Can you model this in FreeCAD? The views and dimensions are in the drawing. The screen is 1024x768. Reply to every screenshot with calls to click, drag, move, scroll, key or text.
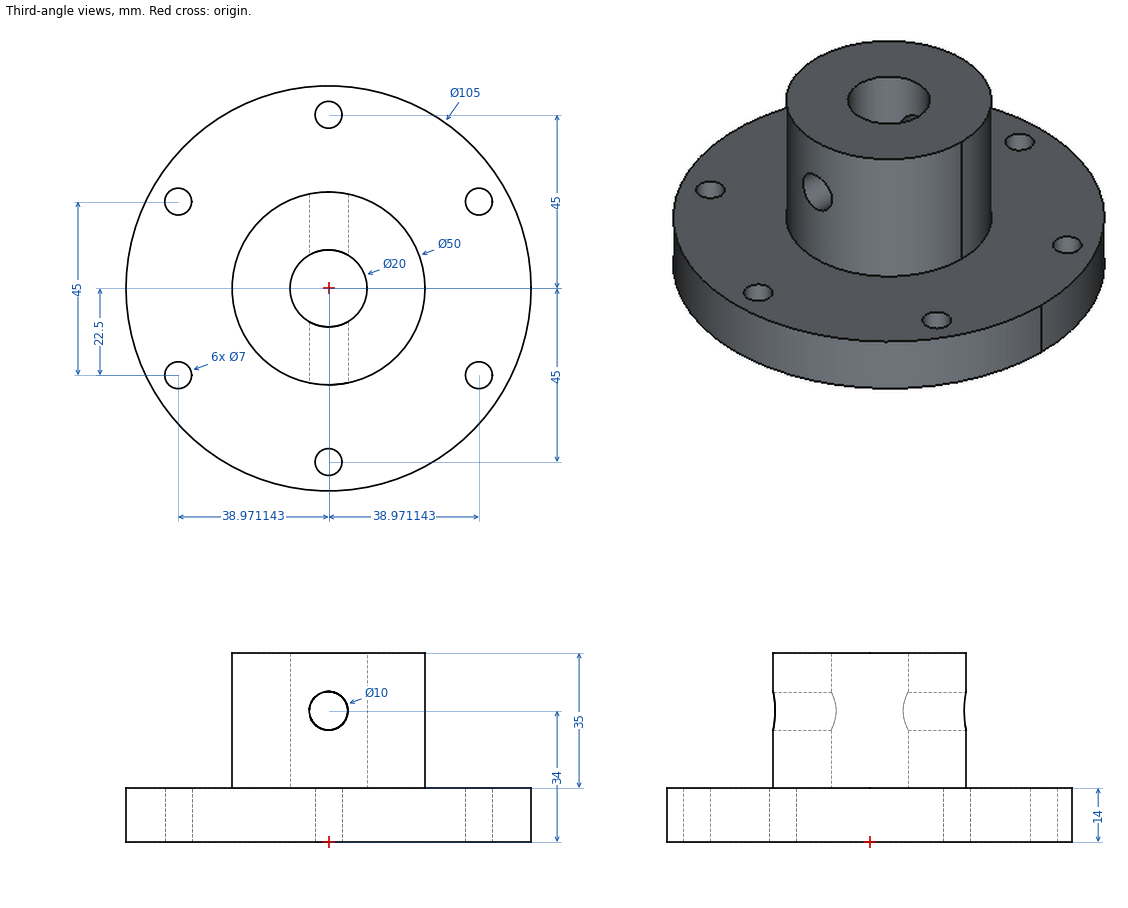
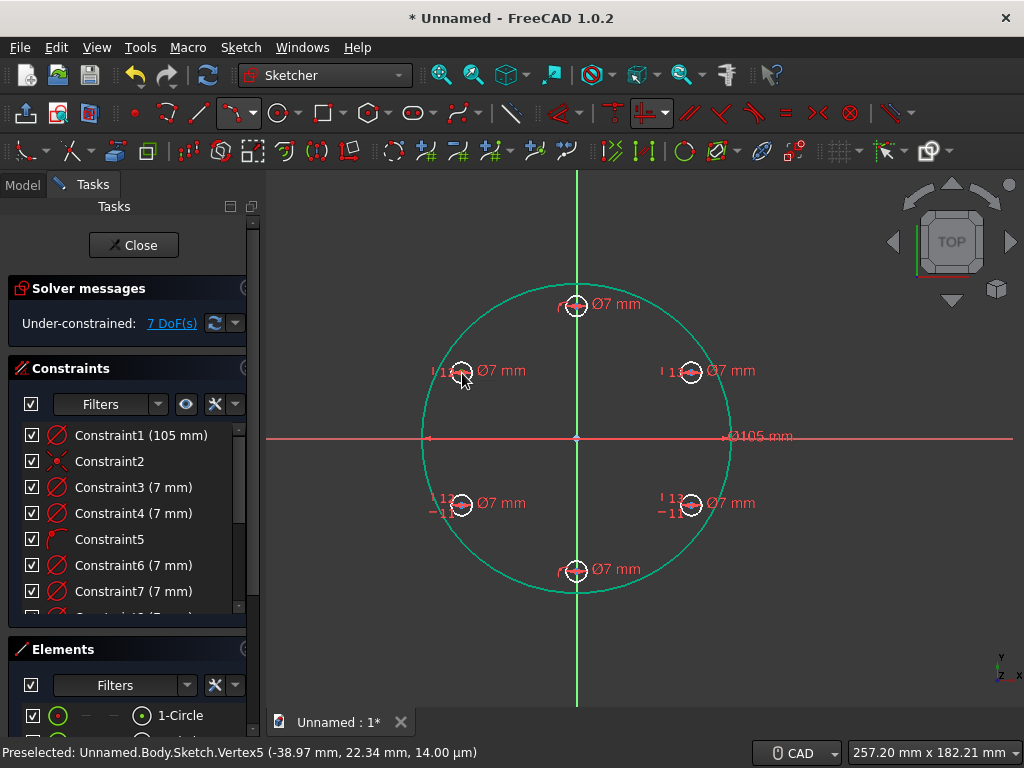
click(691, 373)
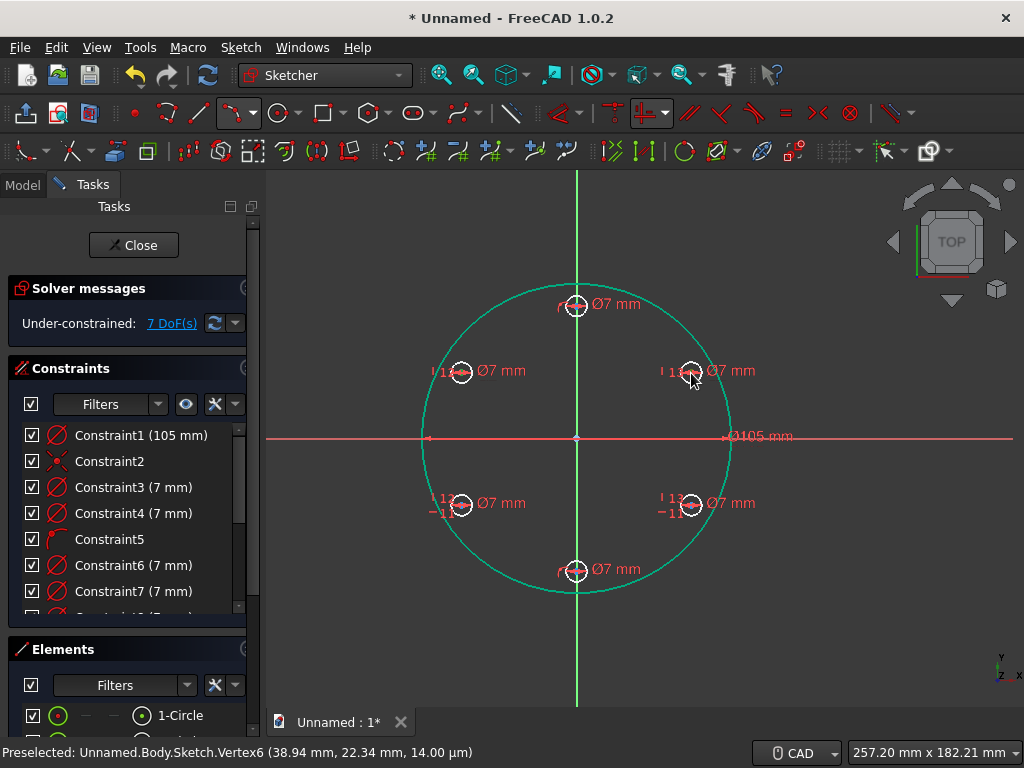
key(h)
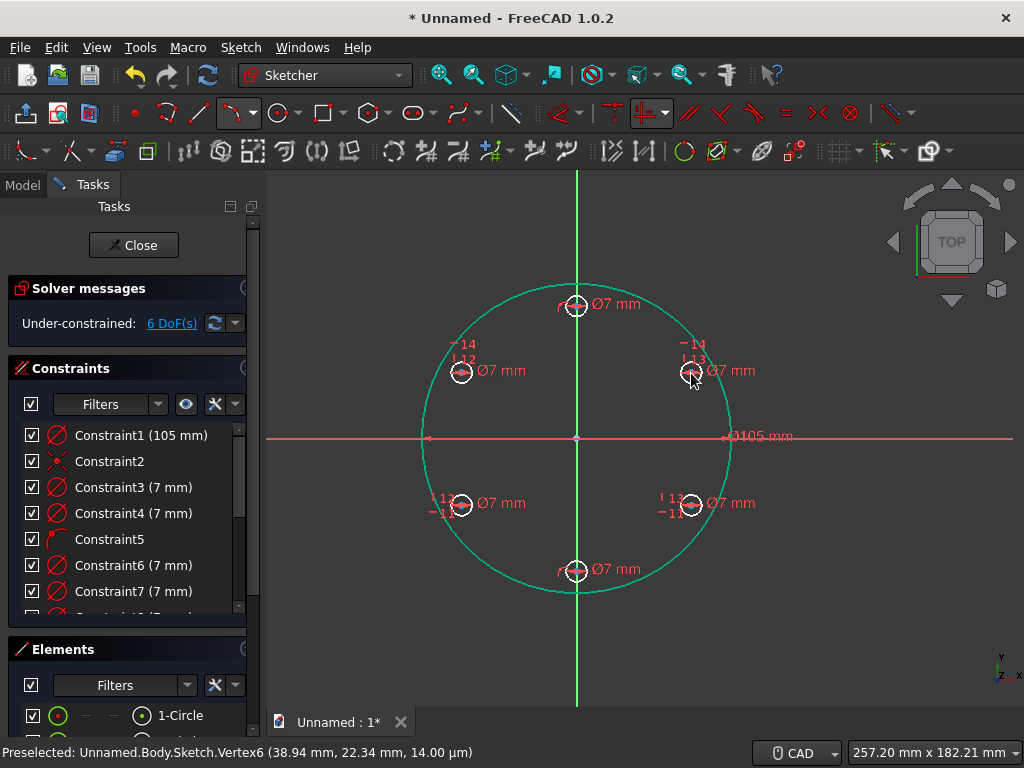
key(d)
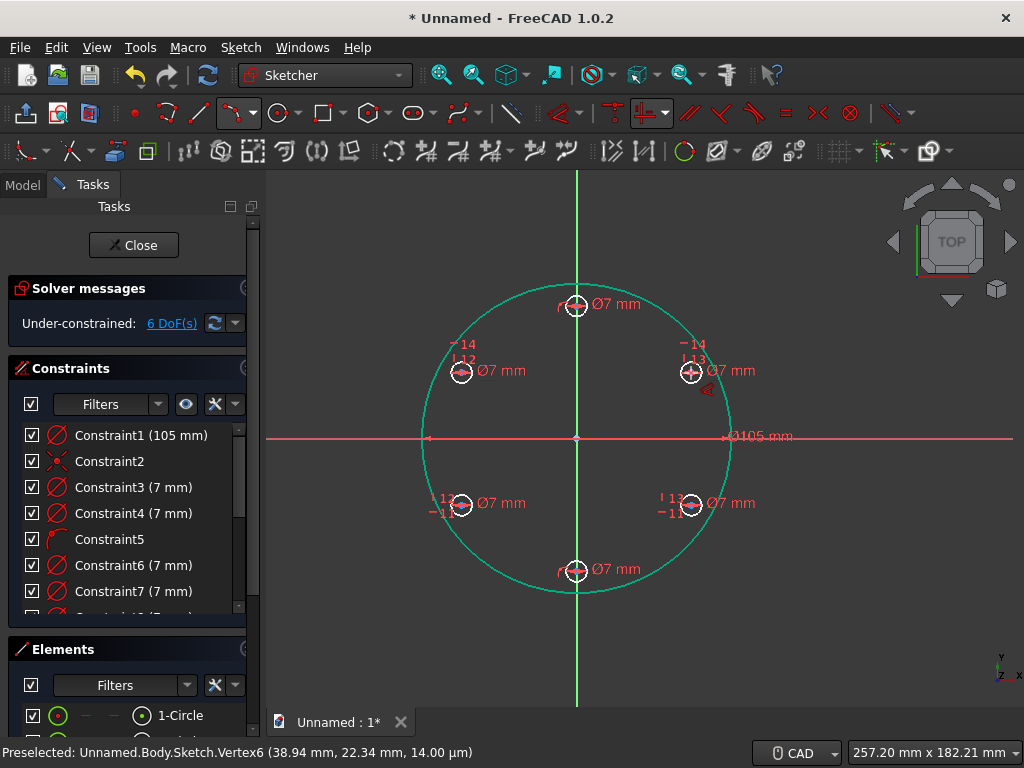
click(577, 571)
click(611, 505)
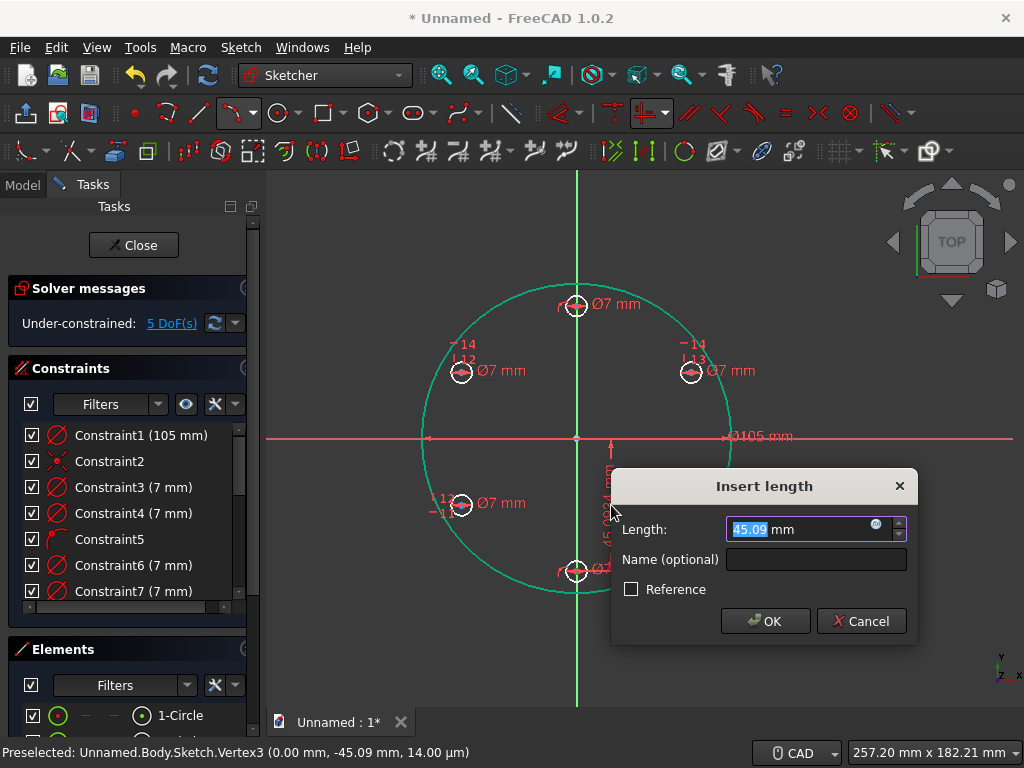
text(45)
key(Return)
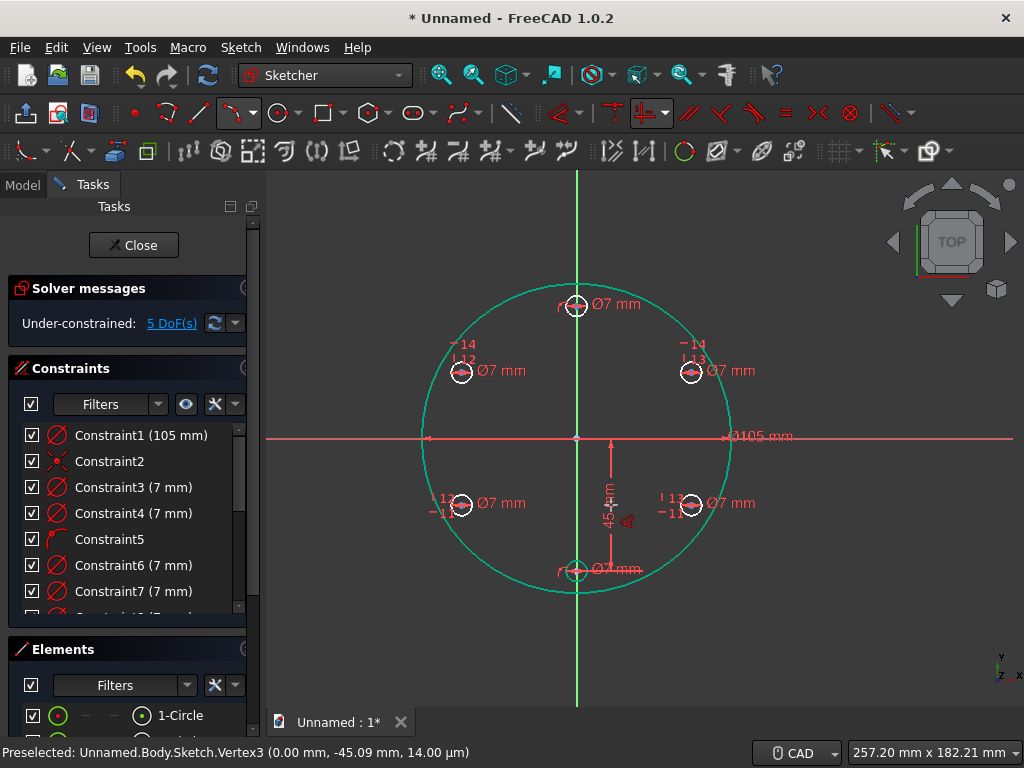
click(577, 306)
click(611, 372)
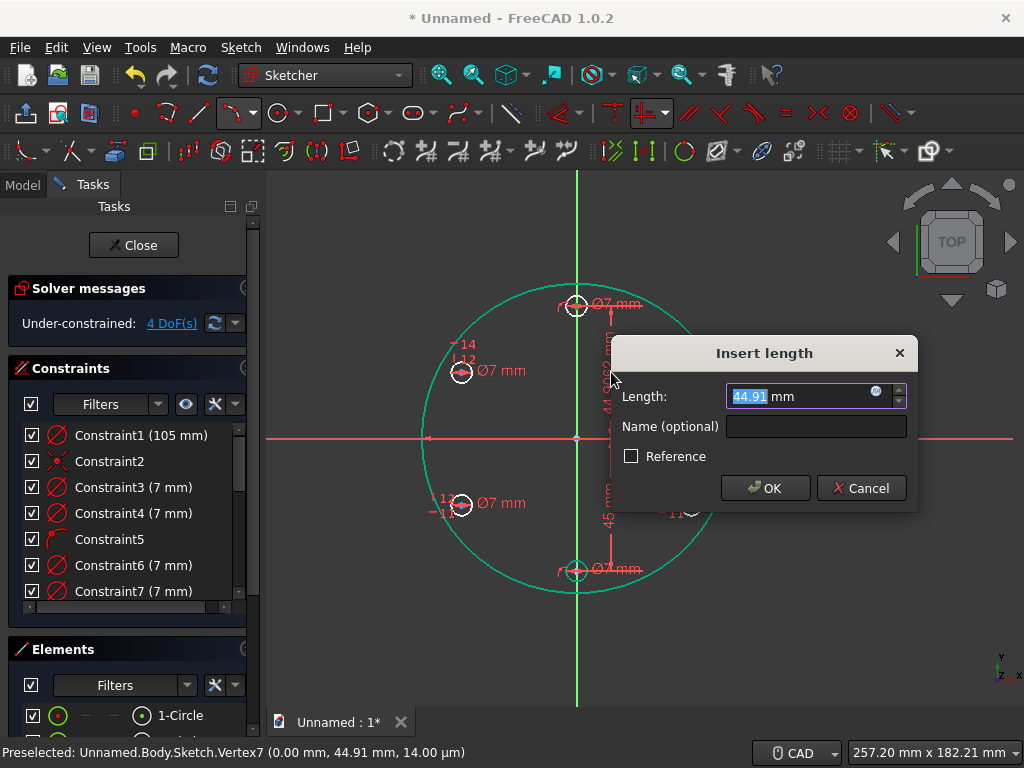
text(45)
key(Return)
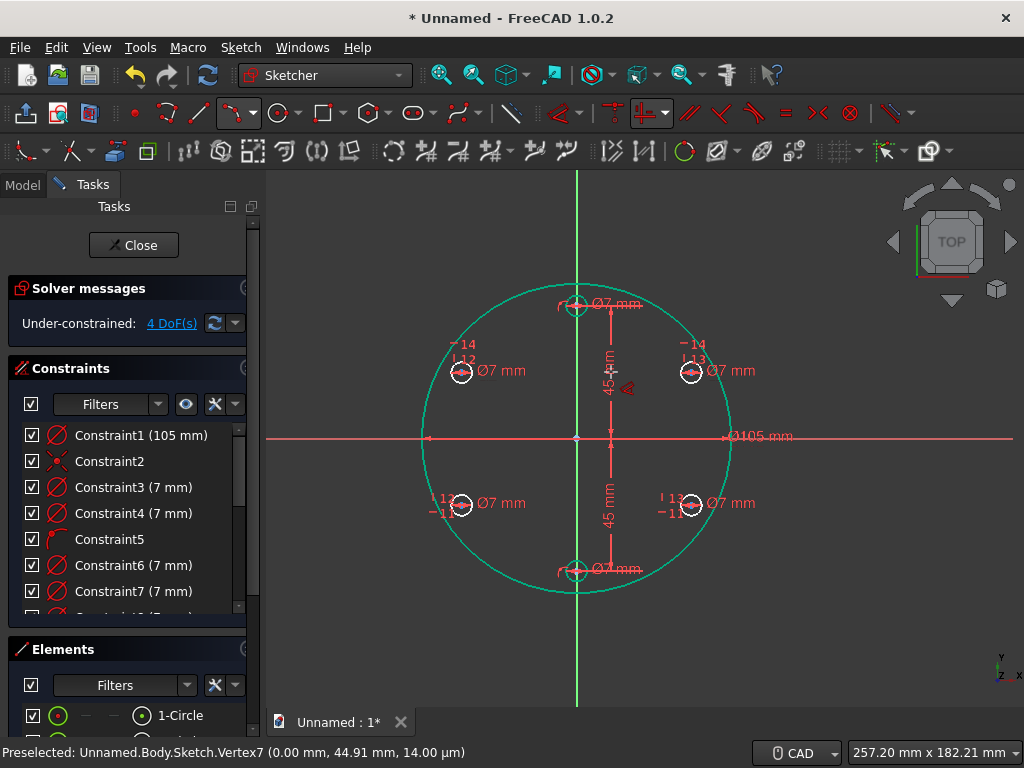
click(462, 505)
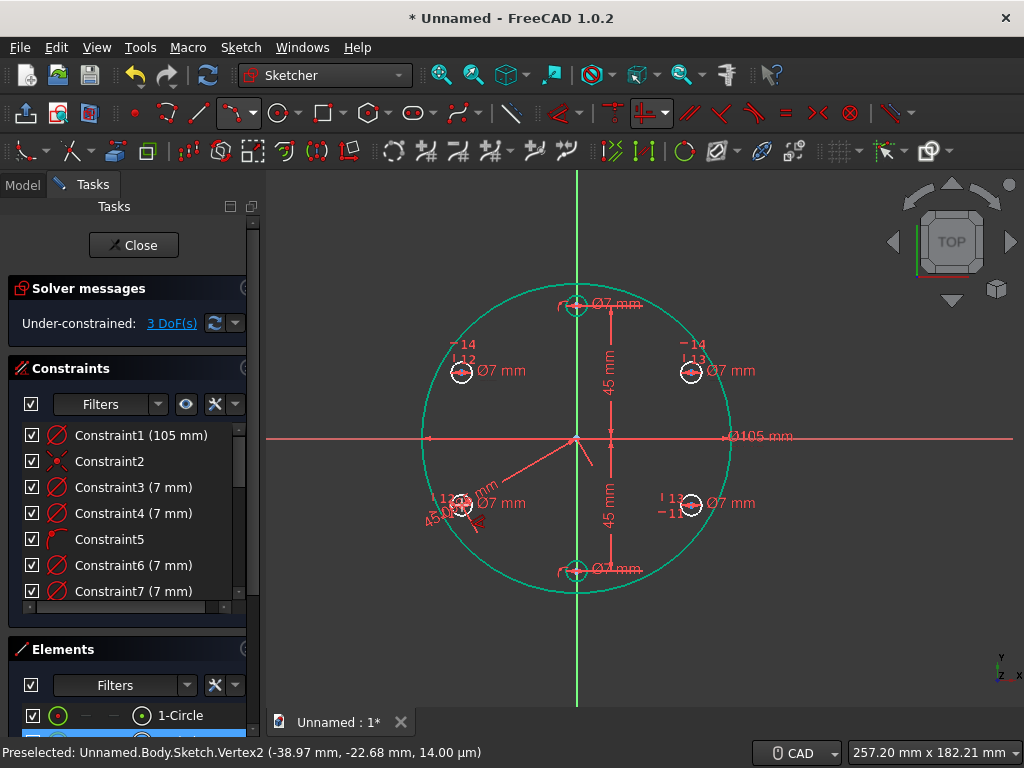
click(462, 373)
click(496, 408)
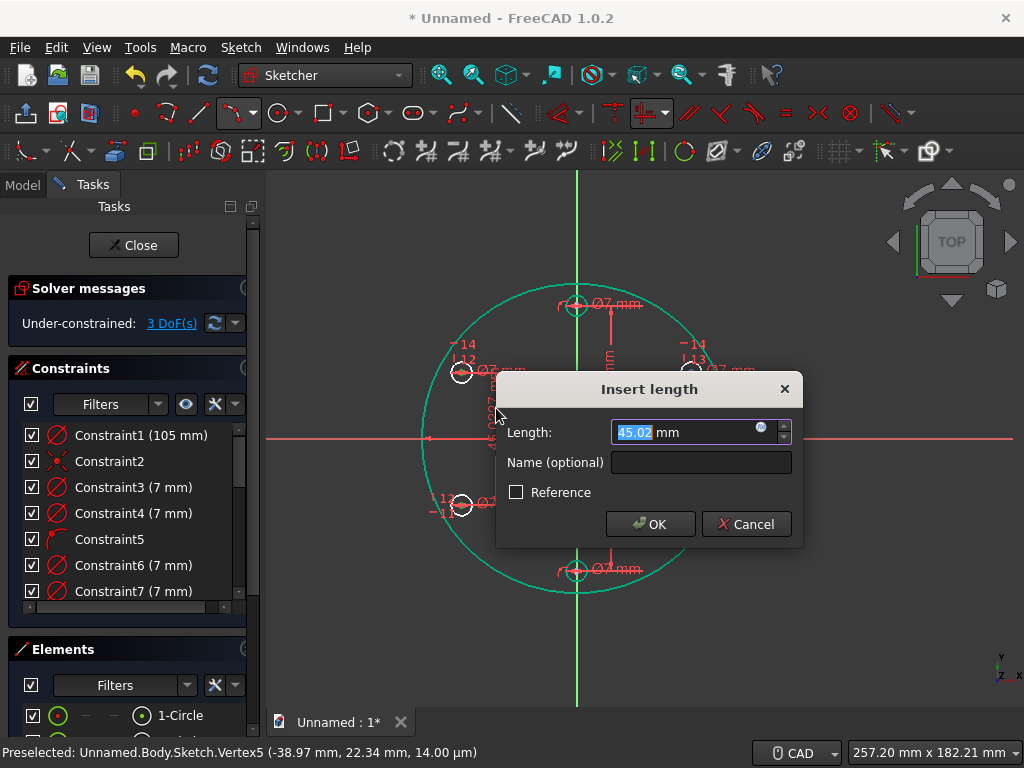
text(45)
key(Return)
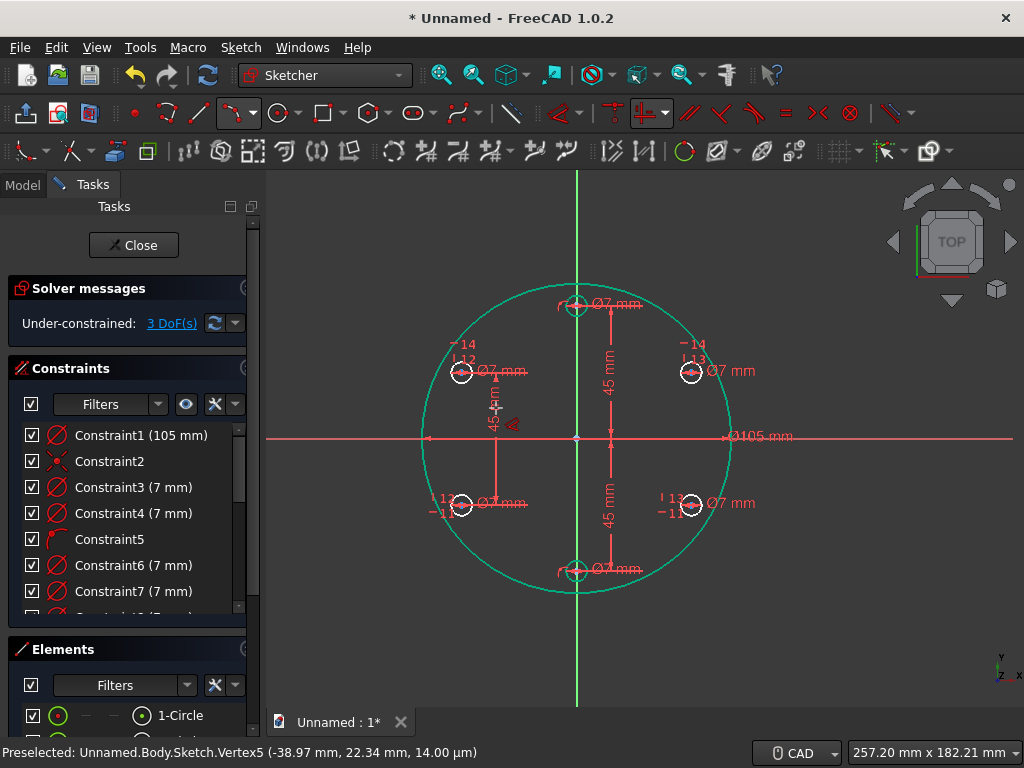
click(462, 505)
click(611, 472)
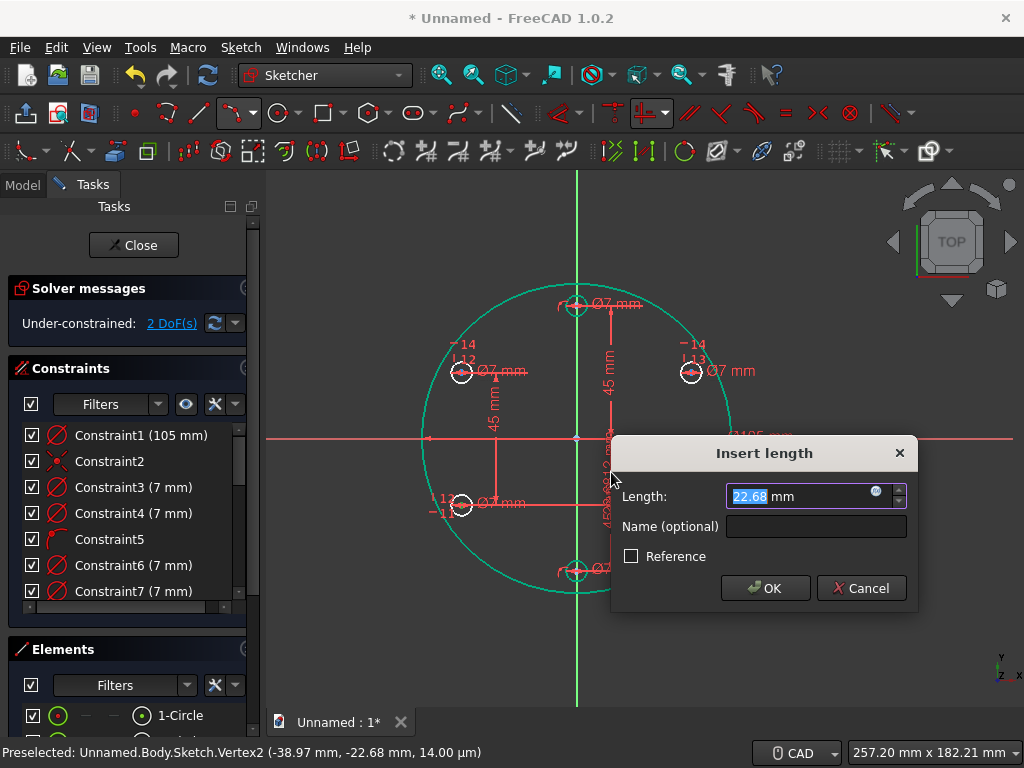
text(22.5)
key(Return)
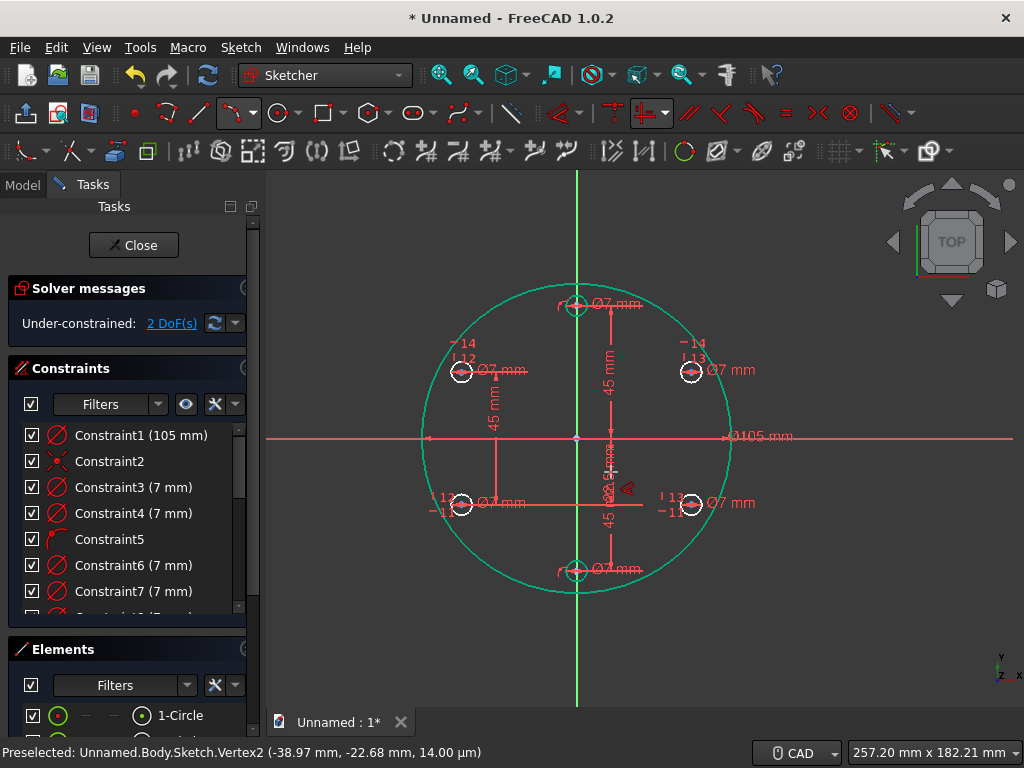
click(462, 505)
click(519, 539)